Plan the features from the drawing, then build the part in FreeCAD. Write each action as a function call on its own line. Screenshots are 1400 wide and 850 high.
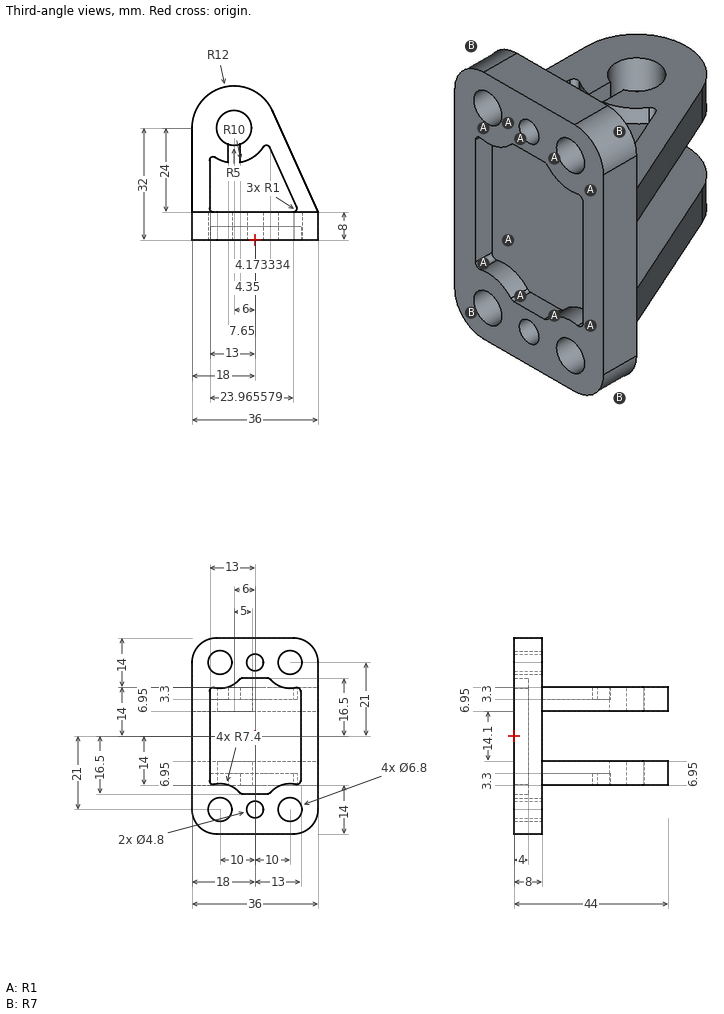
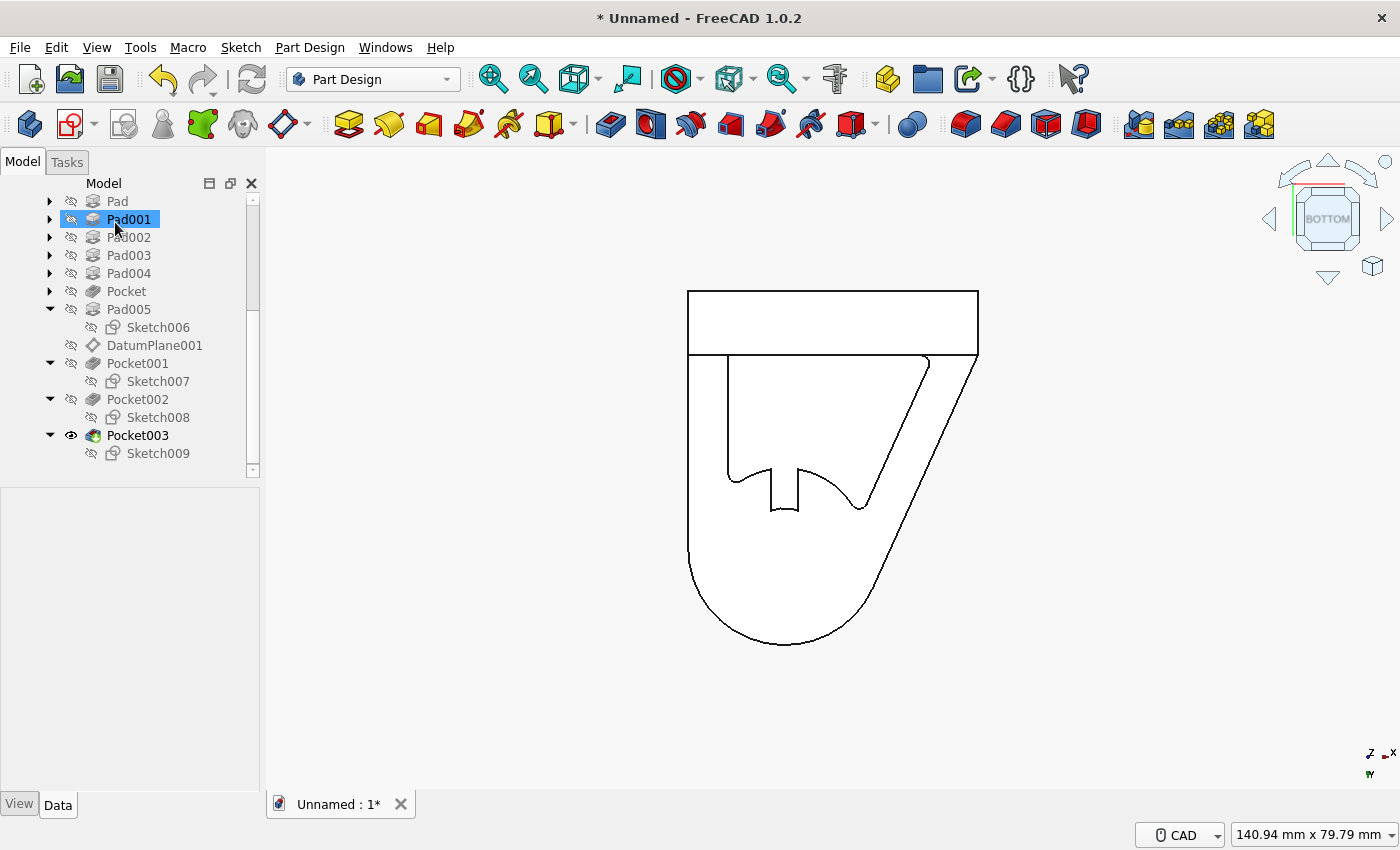
click(70, 124)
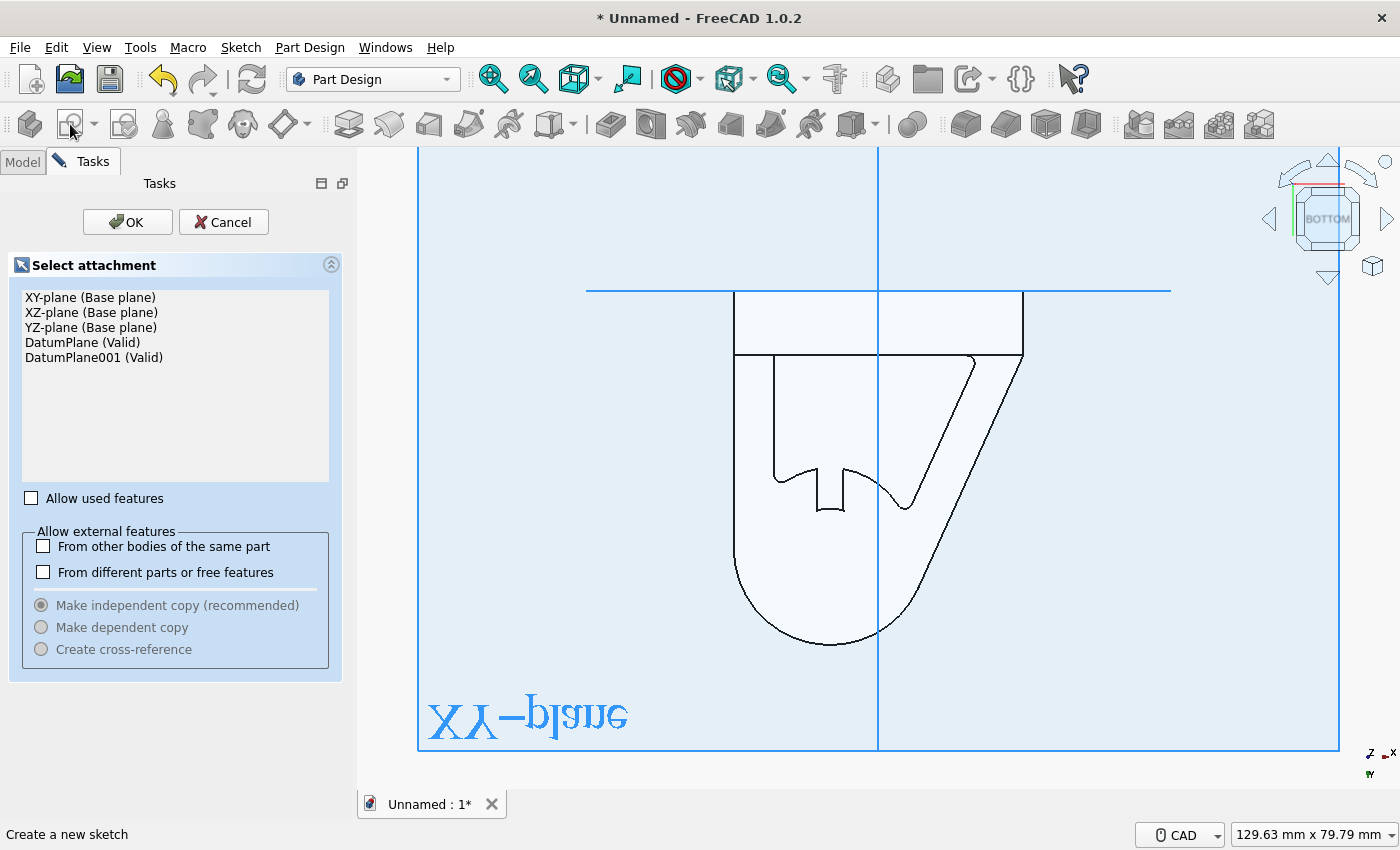
click(82, 312)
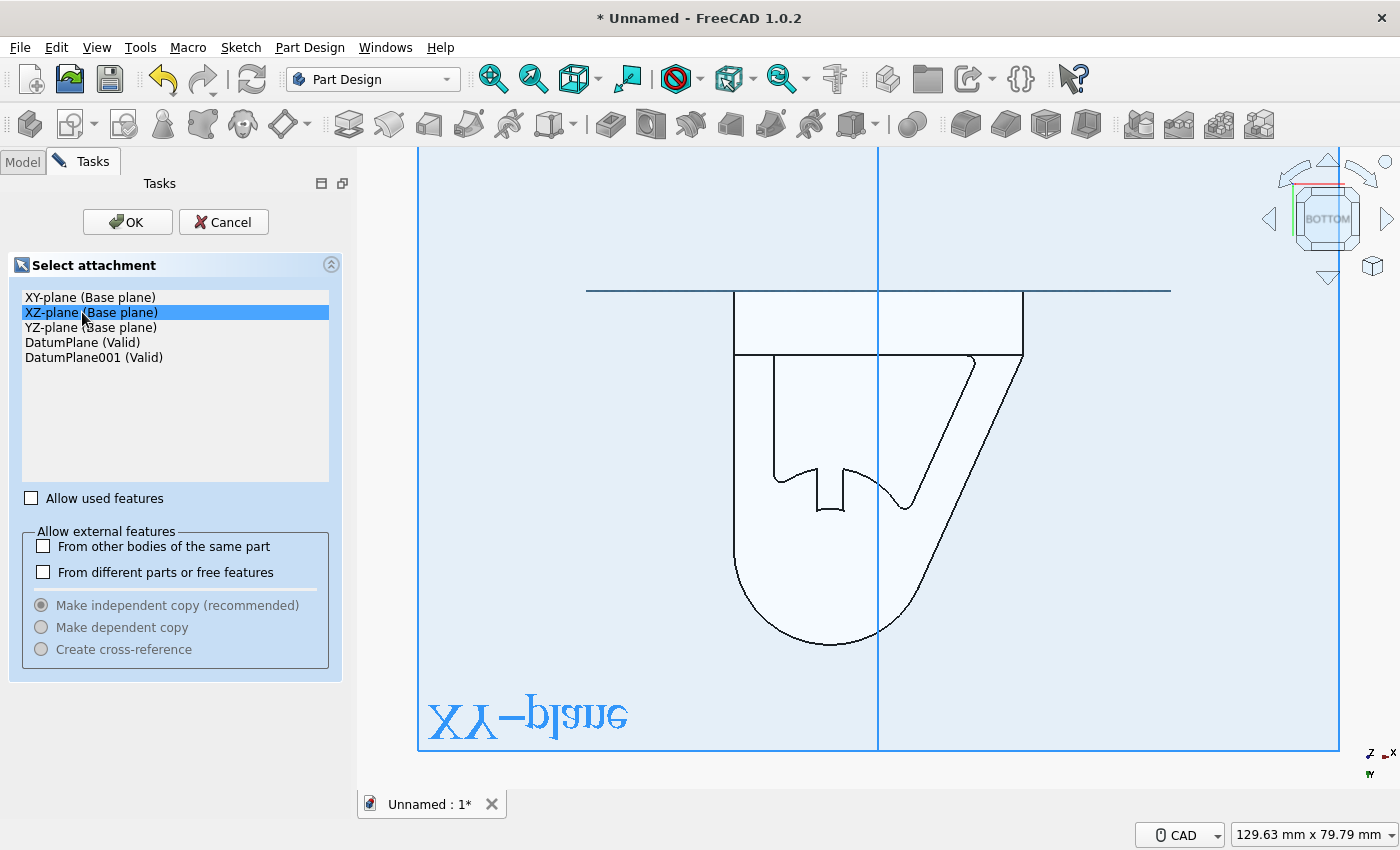
click(128, 222)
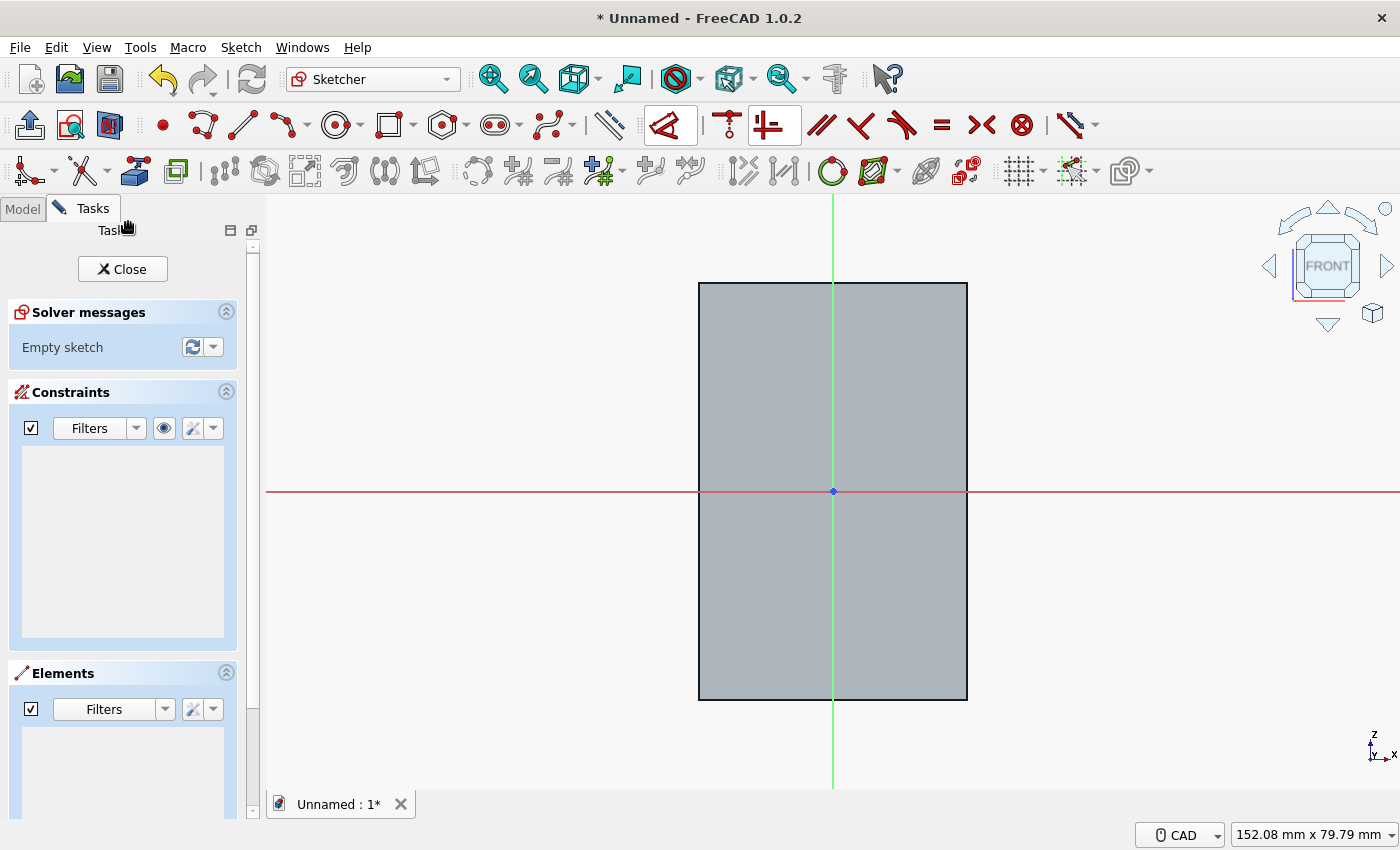
scroll(972, 491, up, 2)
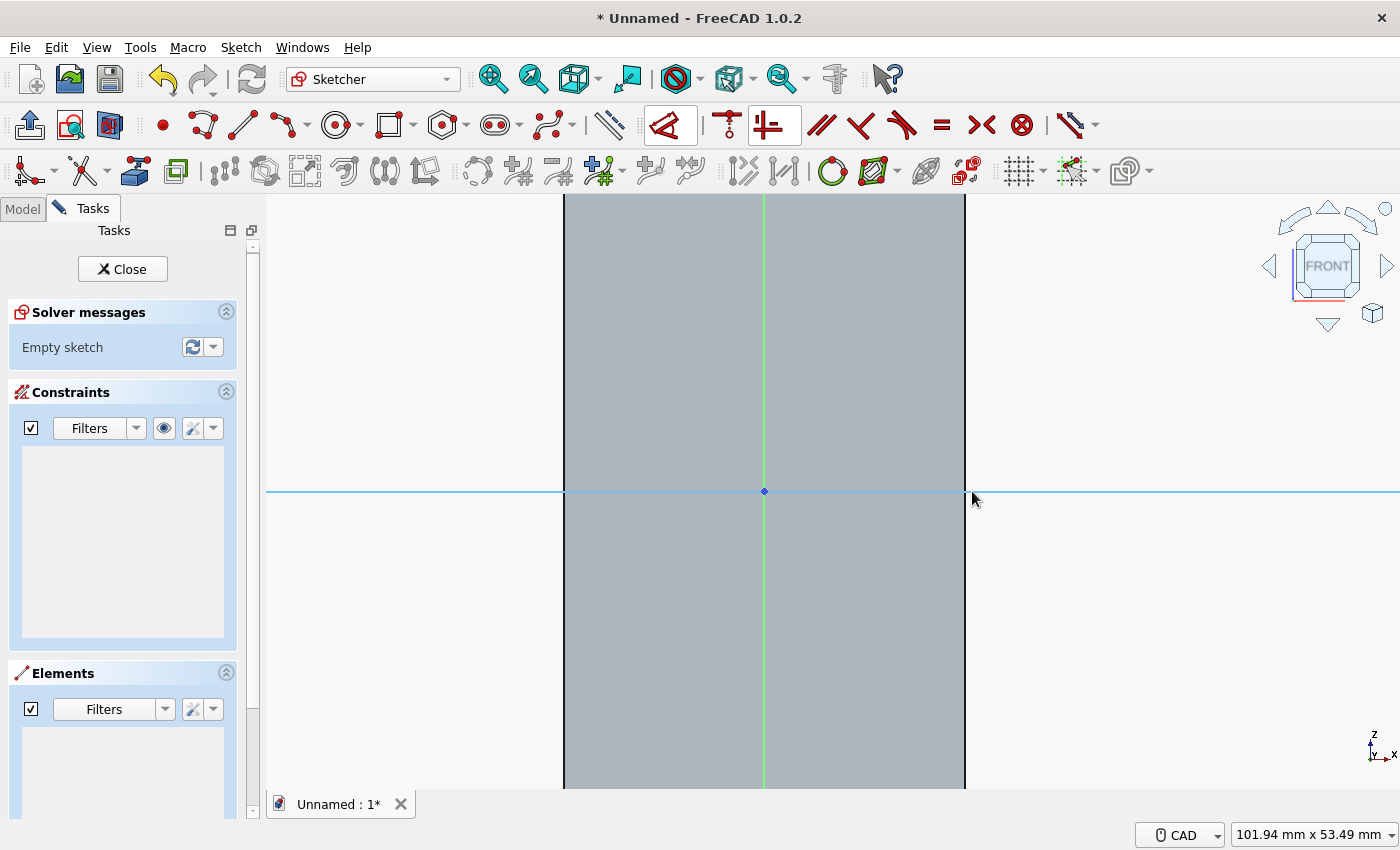
click(244, 126)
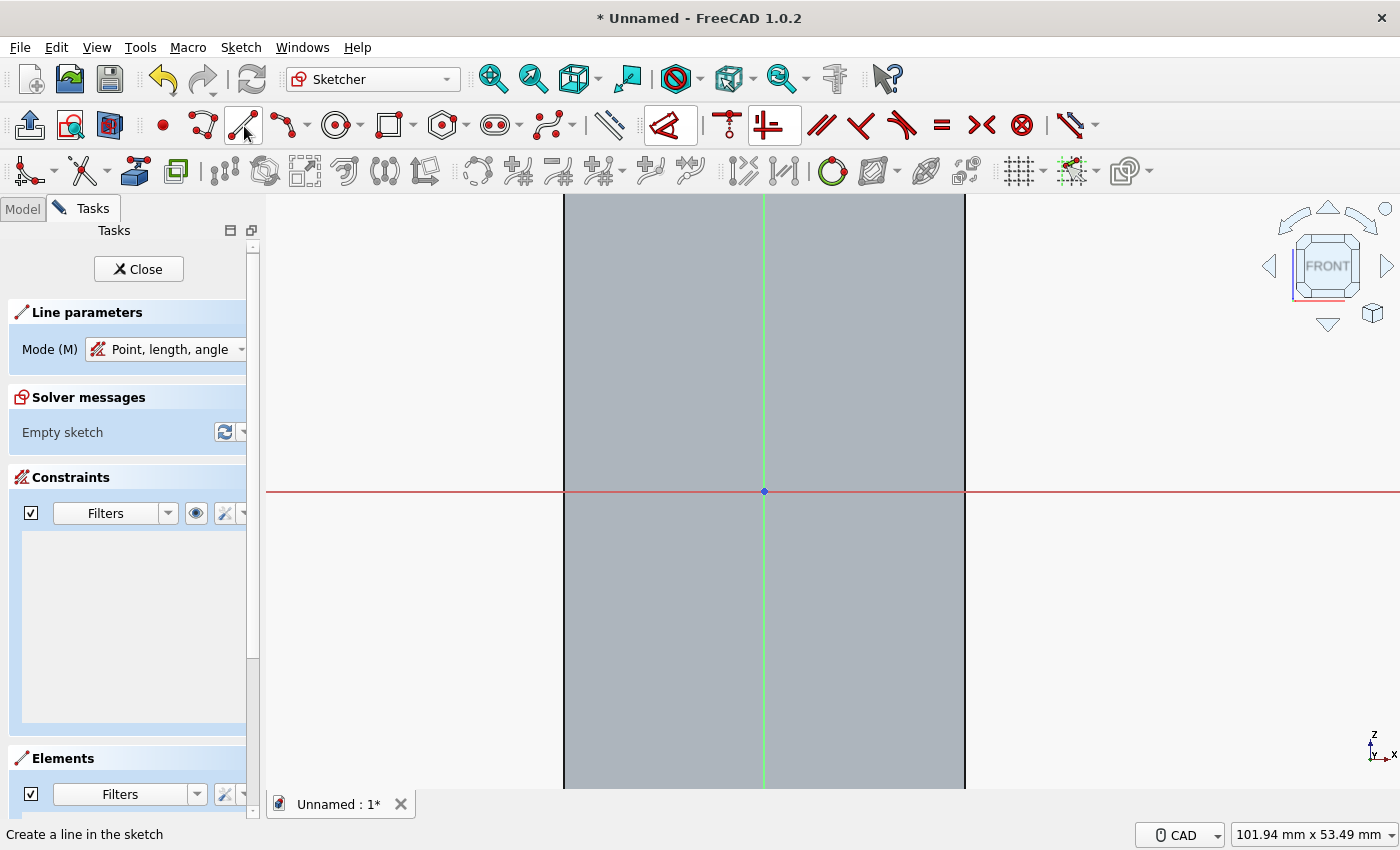
click(620, 333)
click(620, 650)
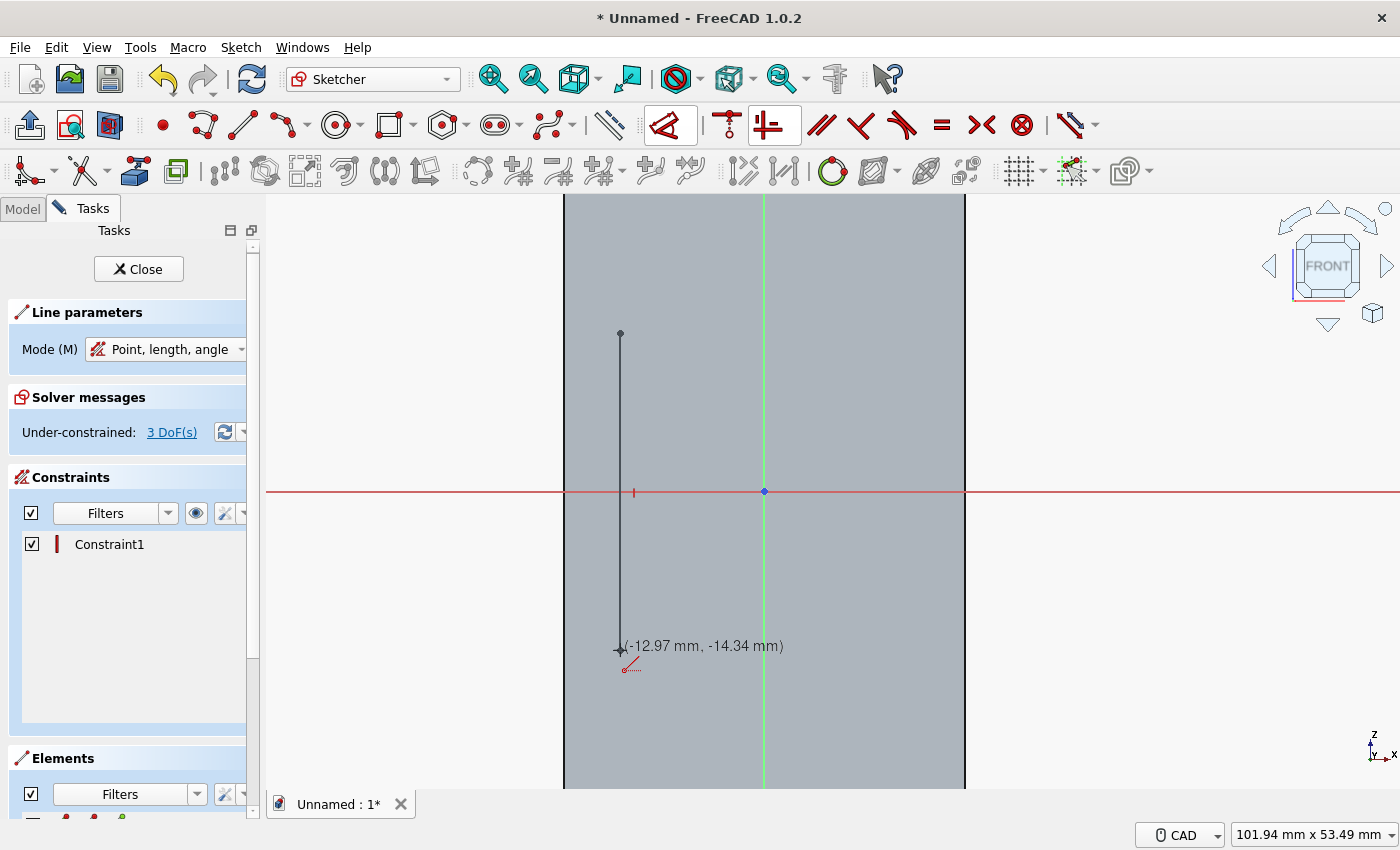
click(718, 675)
click(810, 675)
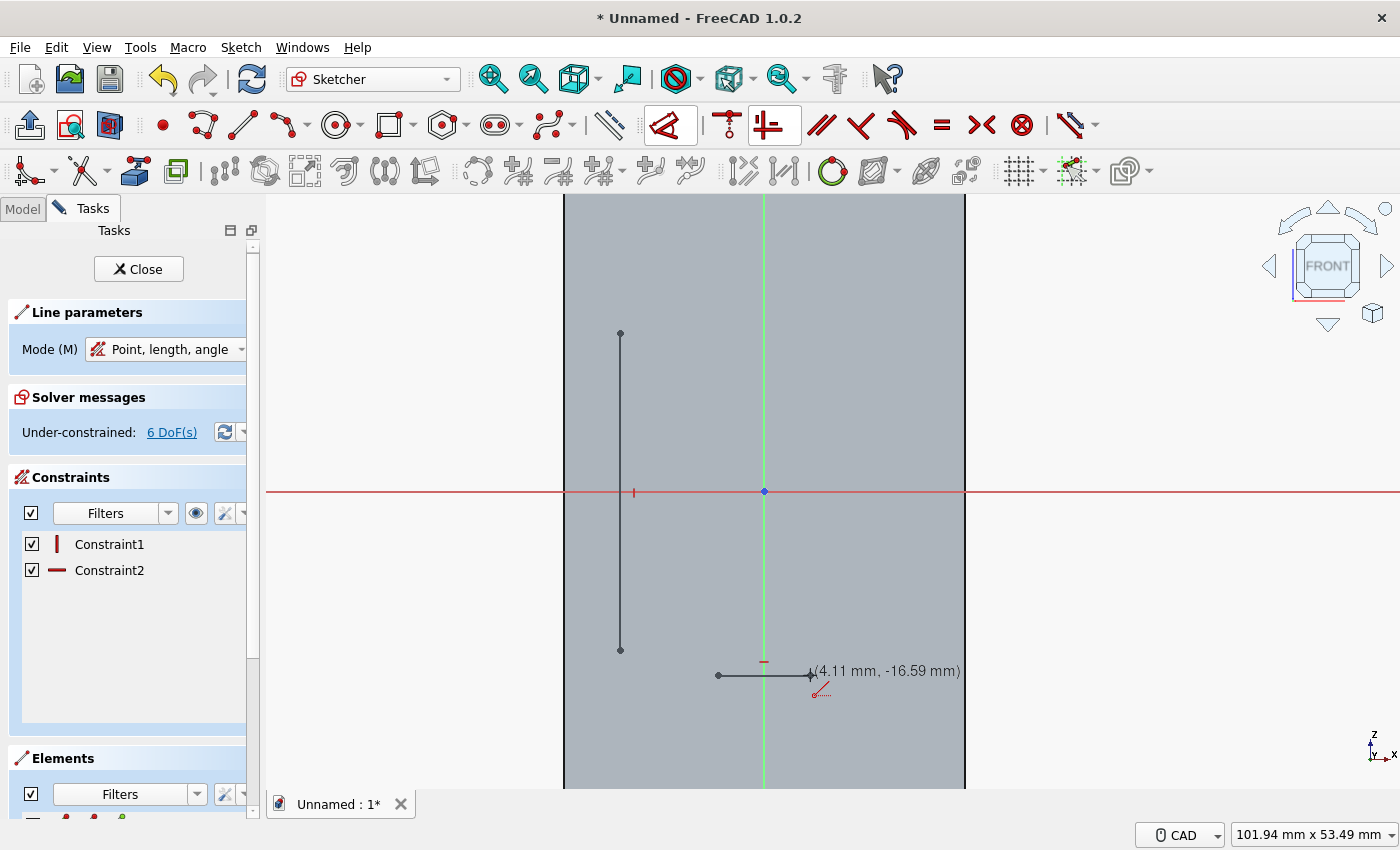
click(909, 650)
click(909, 333)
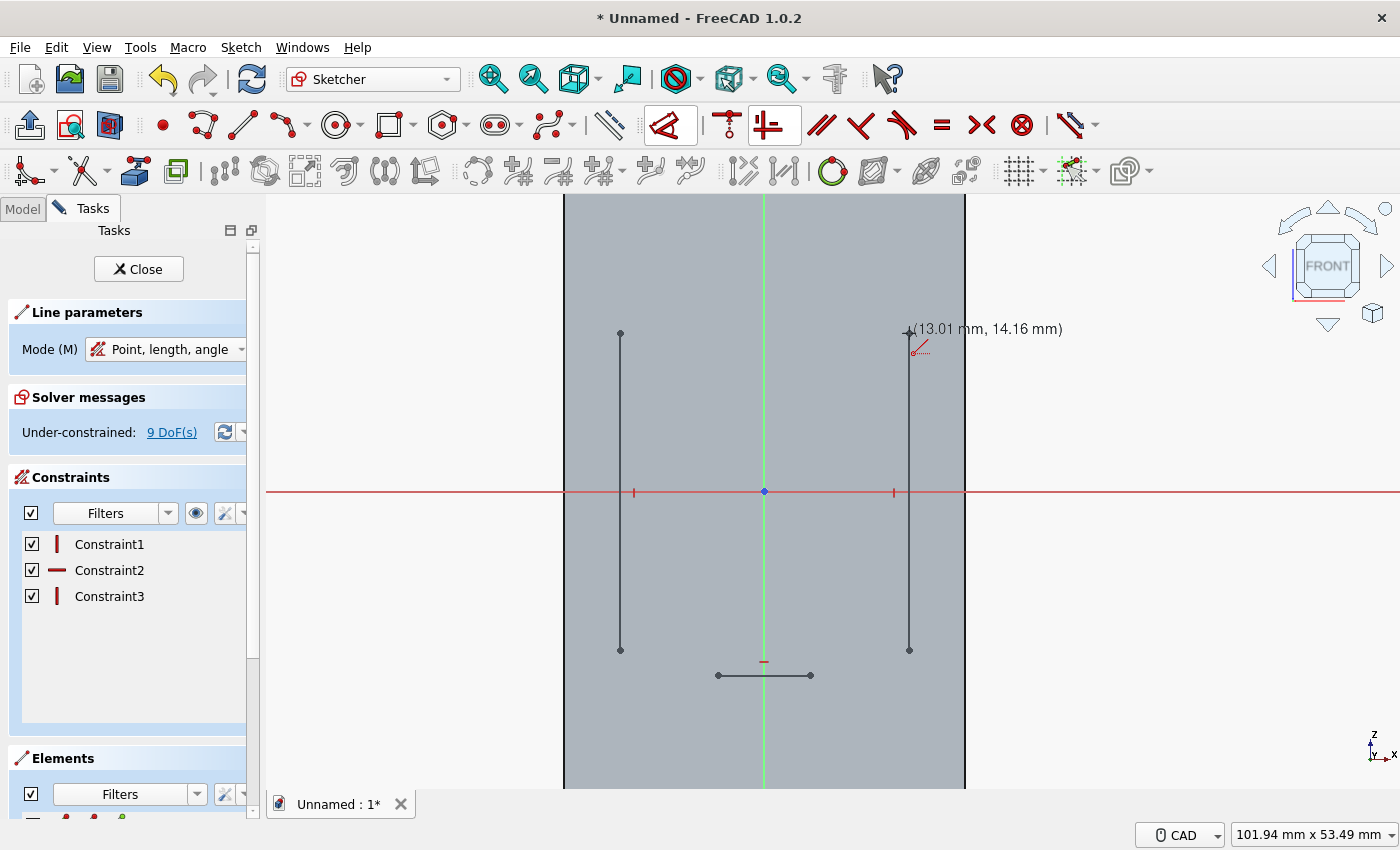
click(810, 308)
click(718, 308)